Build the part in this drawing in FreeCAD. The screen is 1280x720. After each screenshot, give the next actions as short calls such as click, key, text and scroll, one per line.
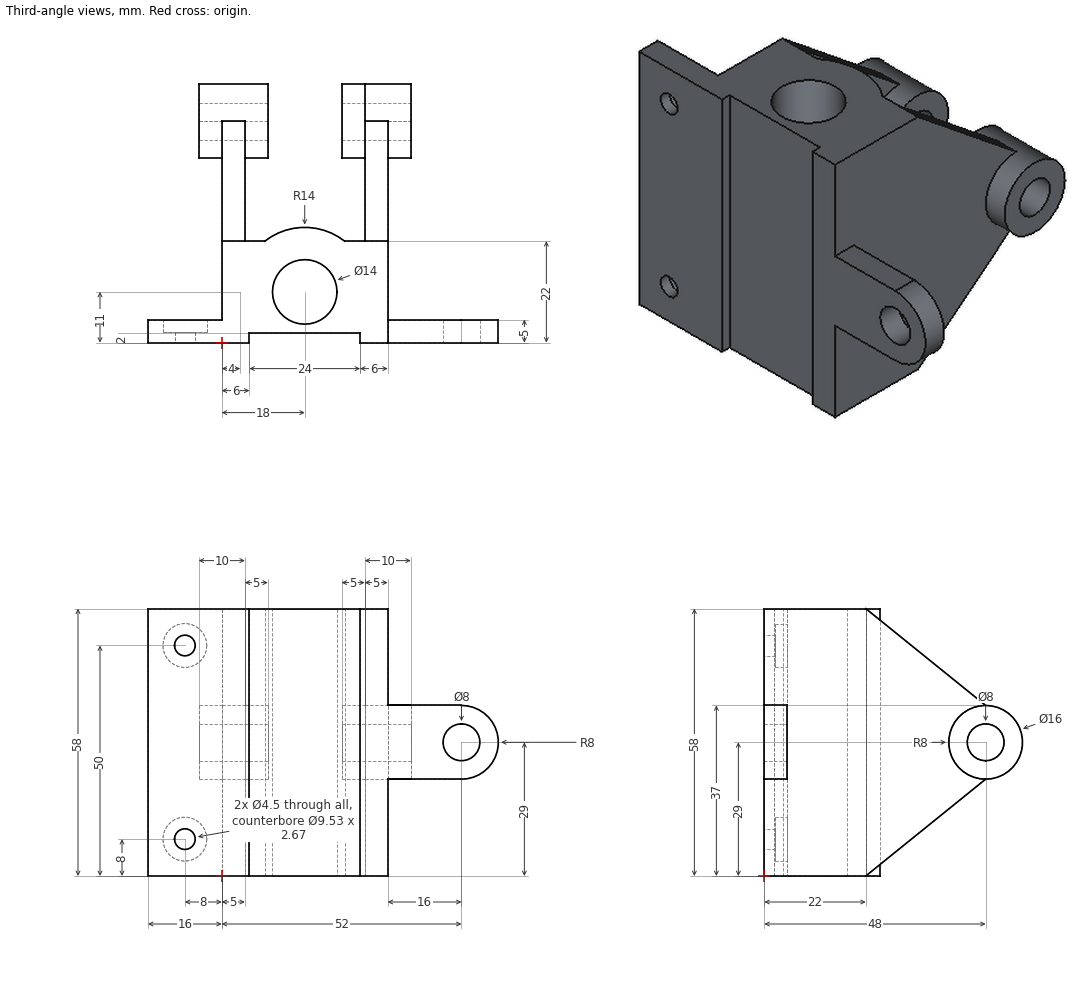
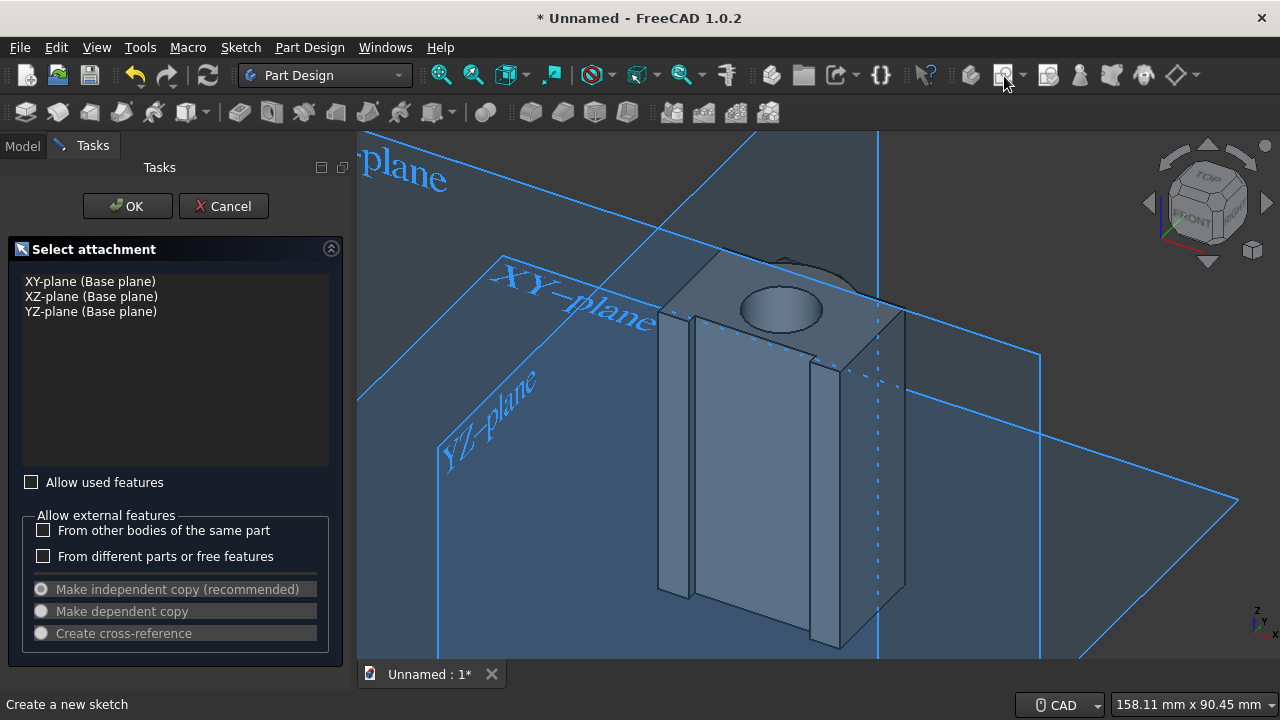
click(82, 312)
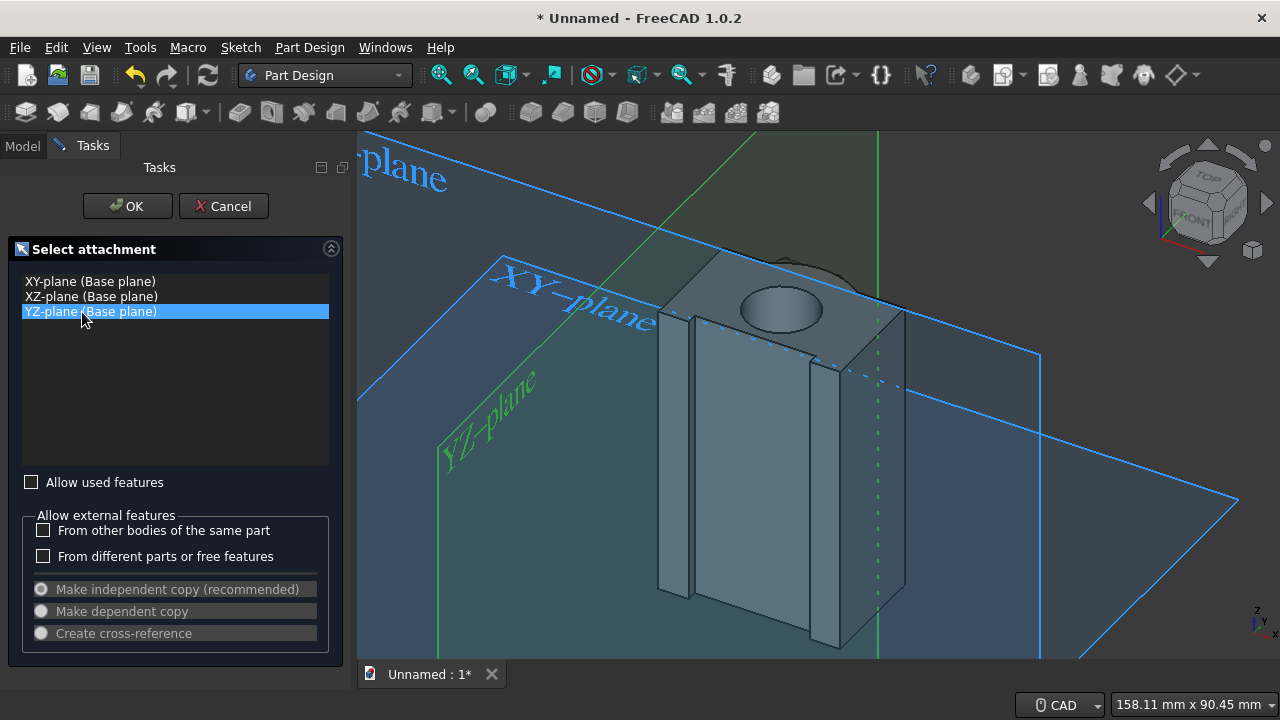
click(128, 206)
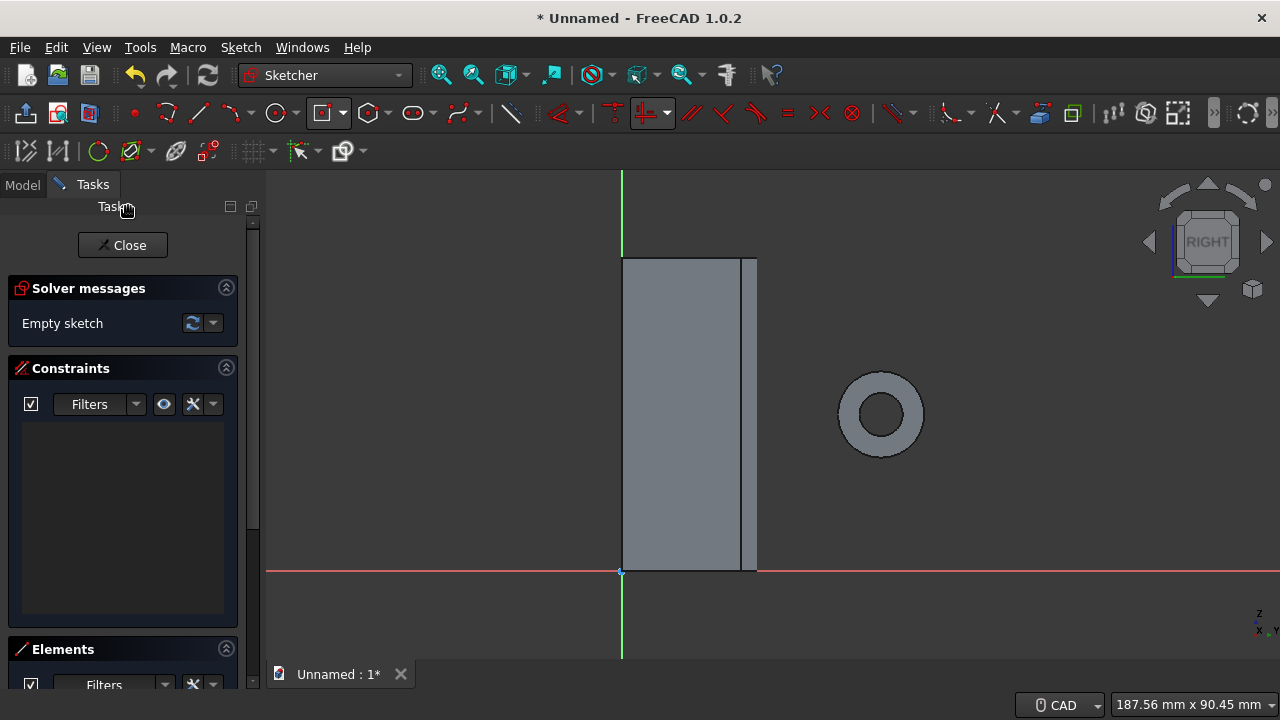
key(q)
key(s)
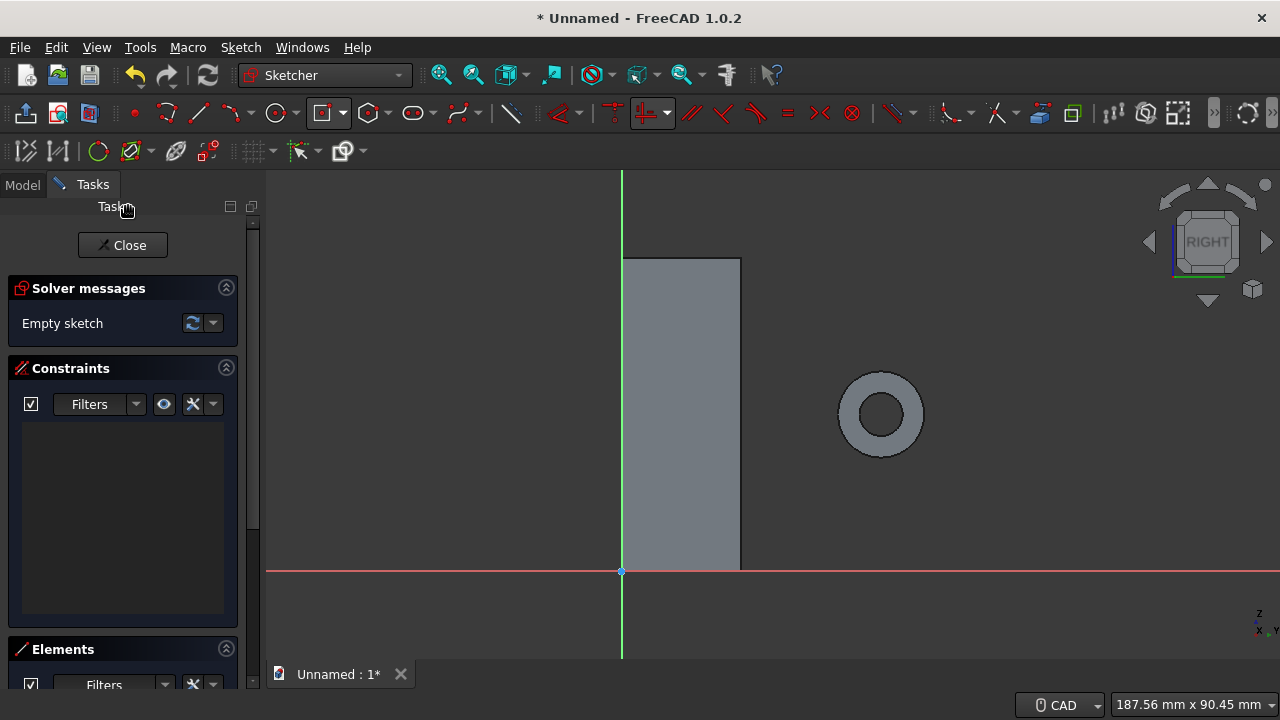
click(168, 114)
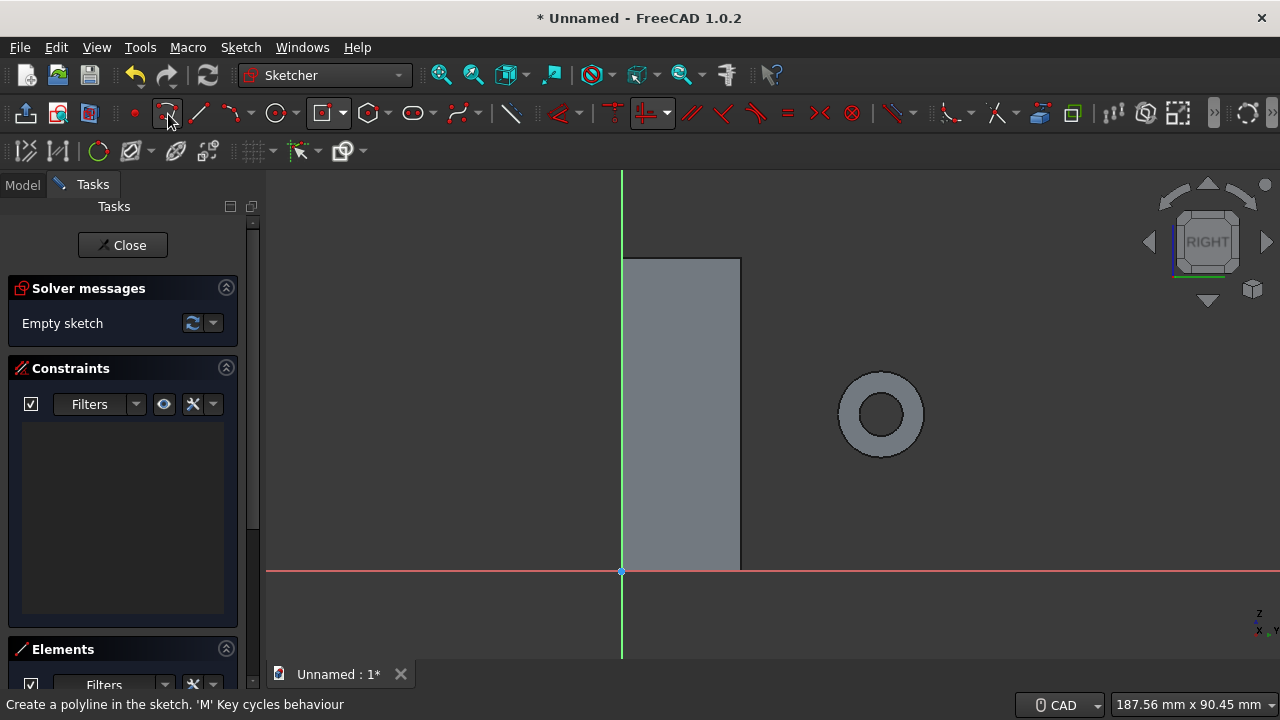
click(881, 371)
click(741, 258)
click(741, 571)
click(881, 458)
right_click(881, 458)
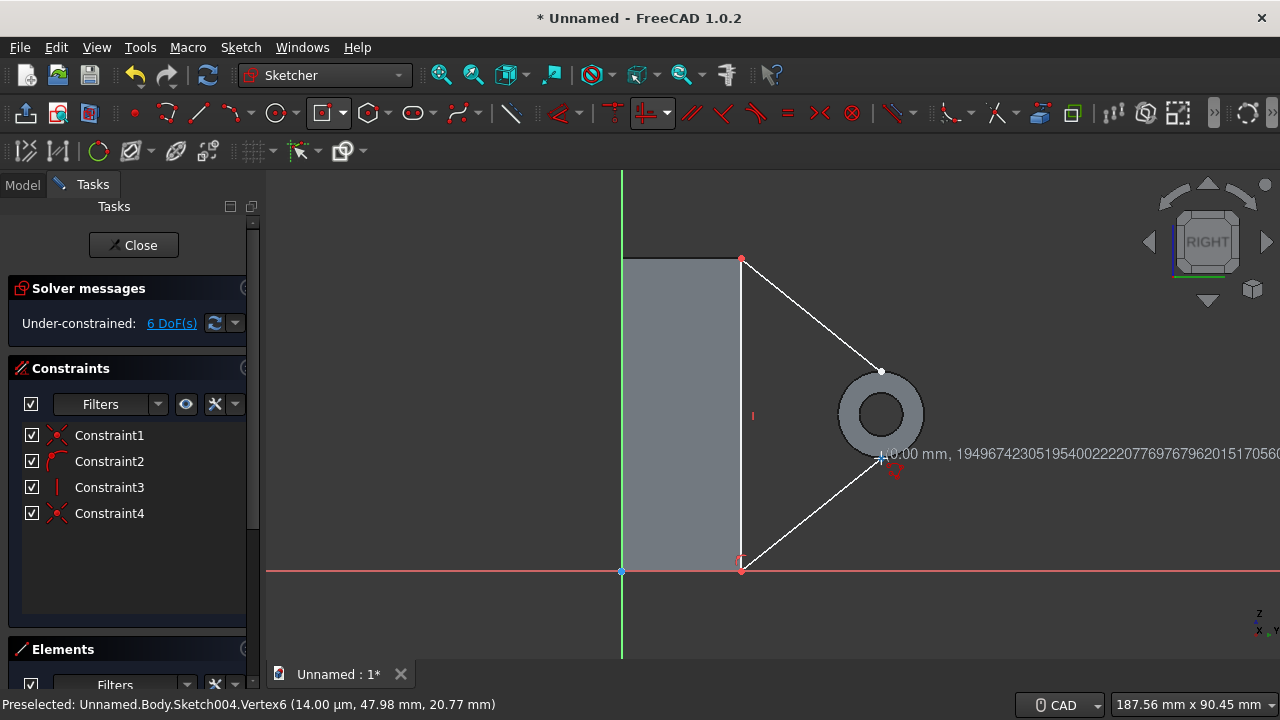
click(232, 114)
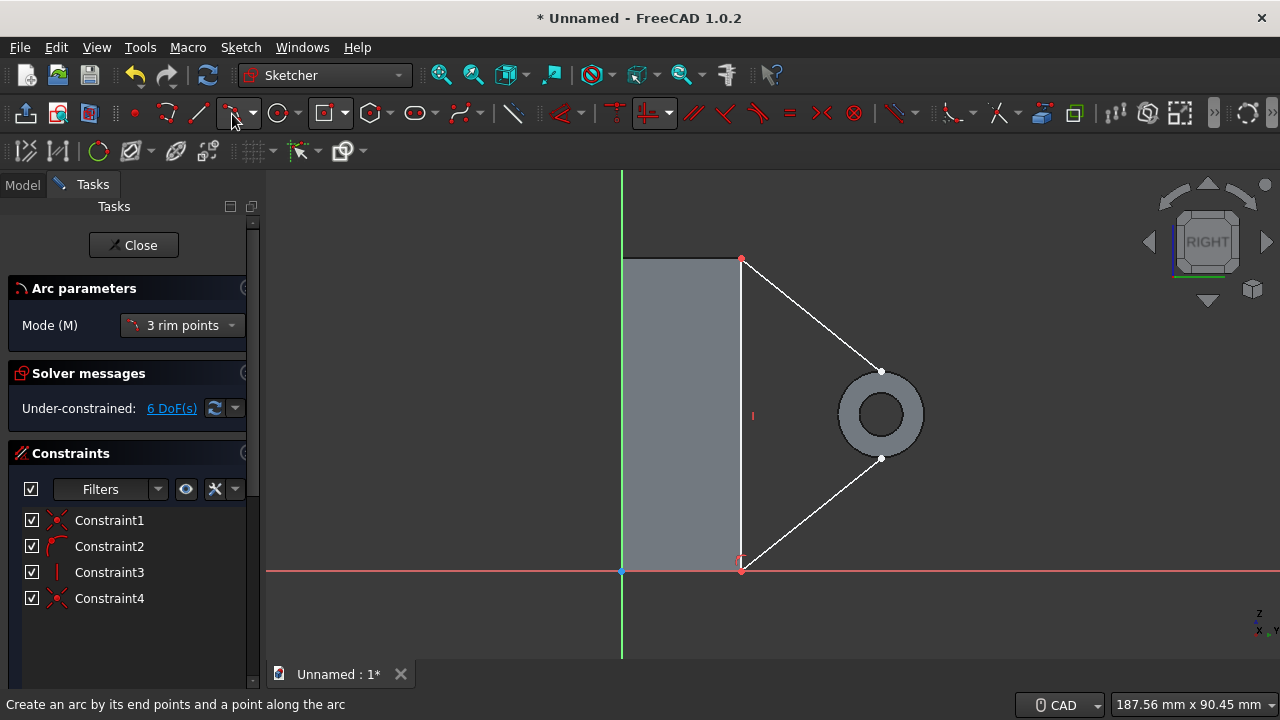
click(881, 459)
click(881, 372)
click(838, 414)
key(Escape)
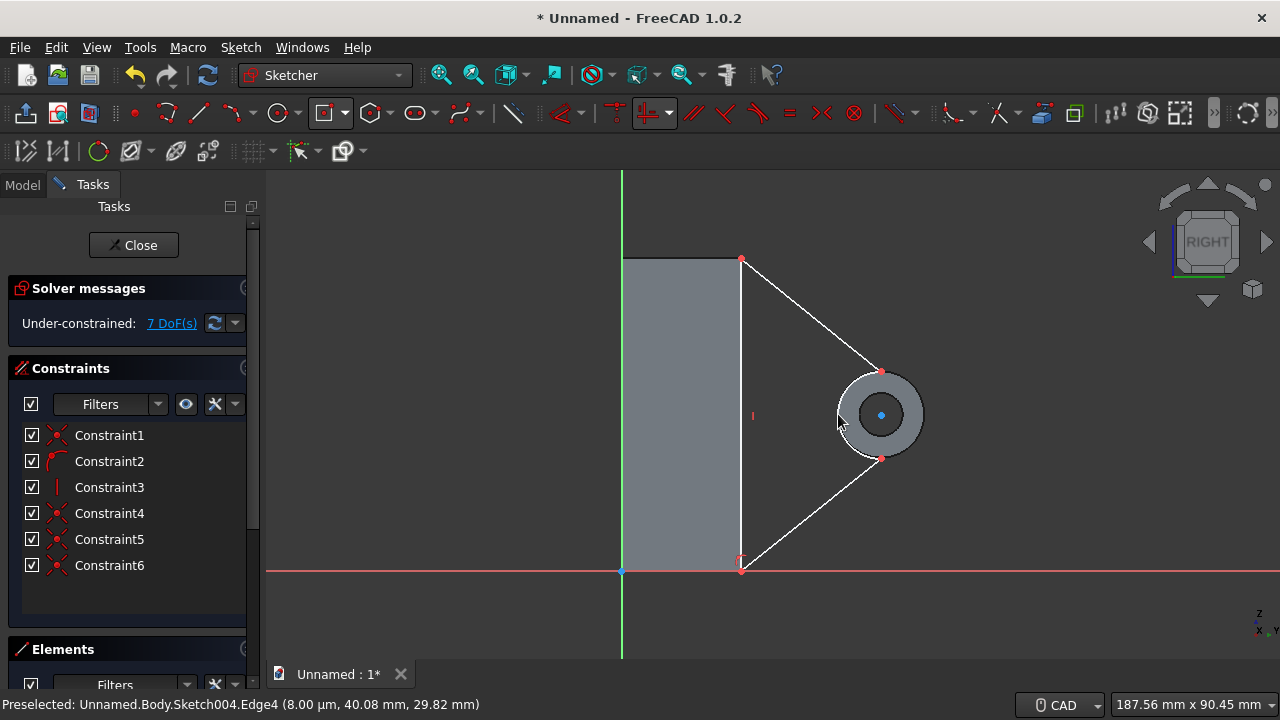
click(560, 114)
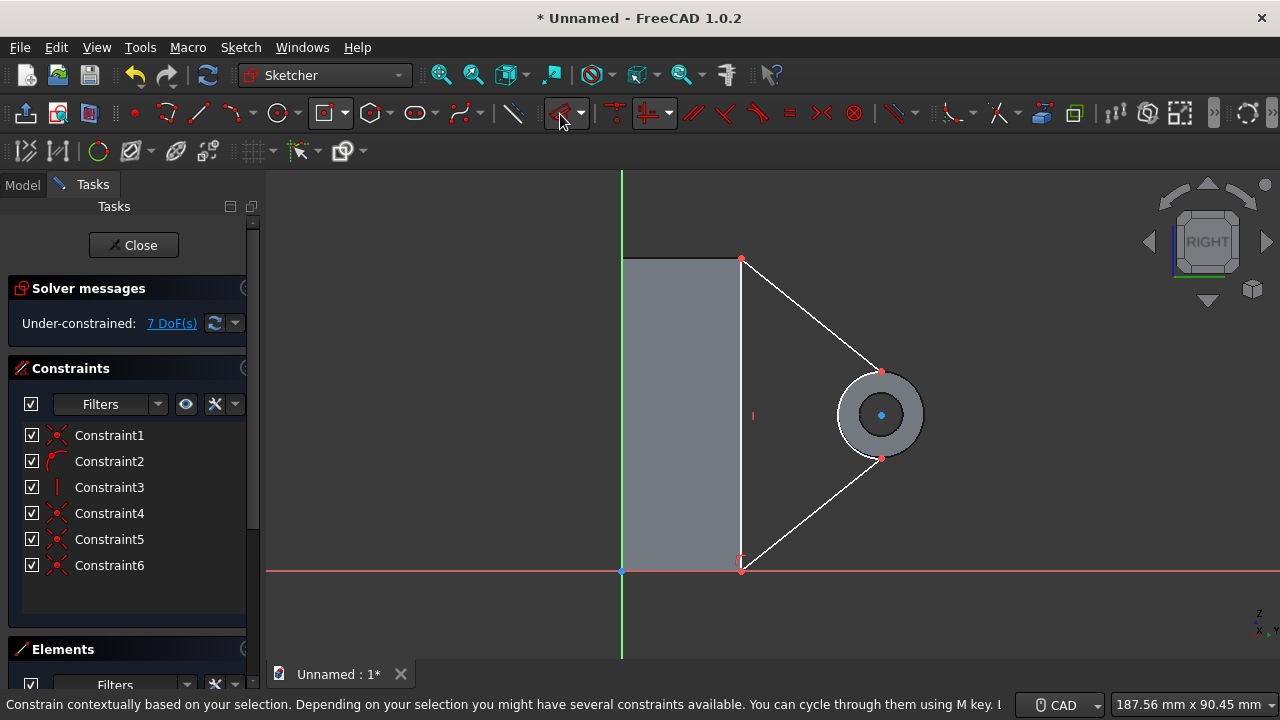
click(846, 390)
click(820, 371)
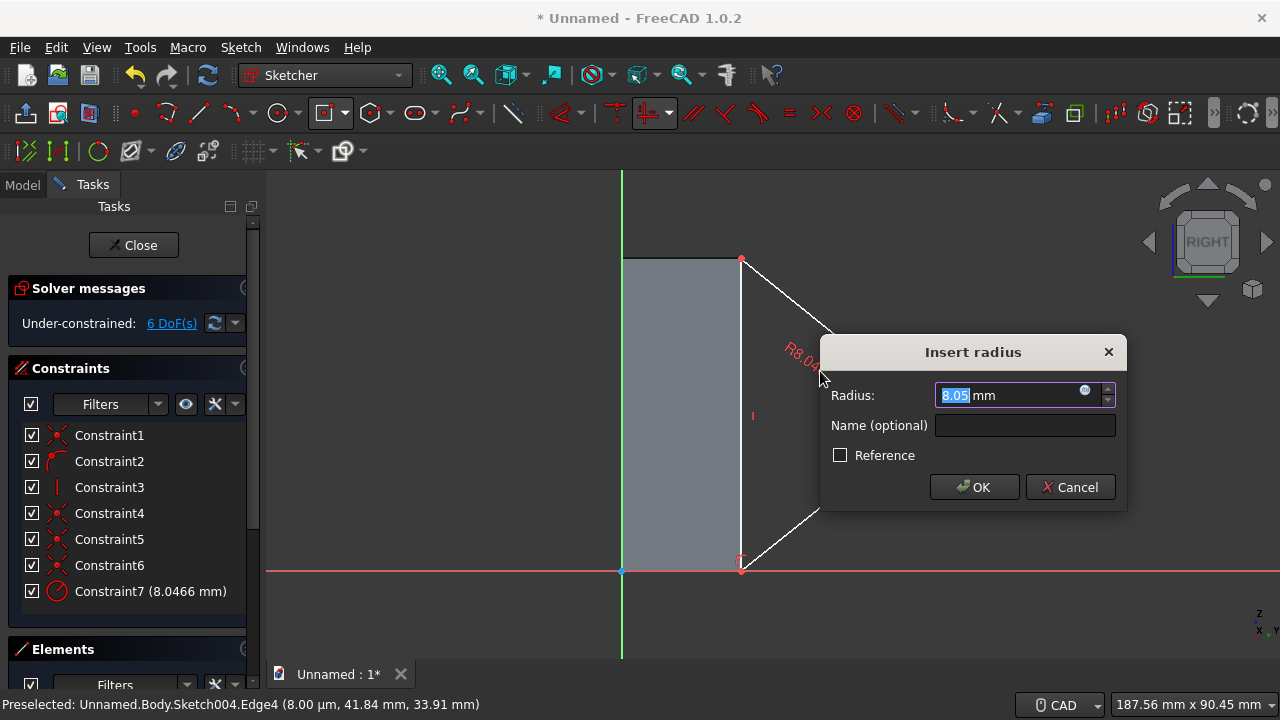
text(8)
key(Return)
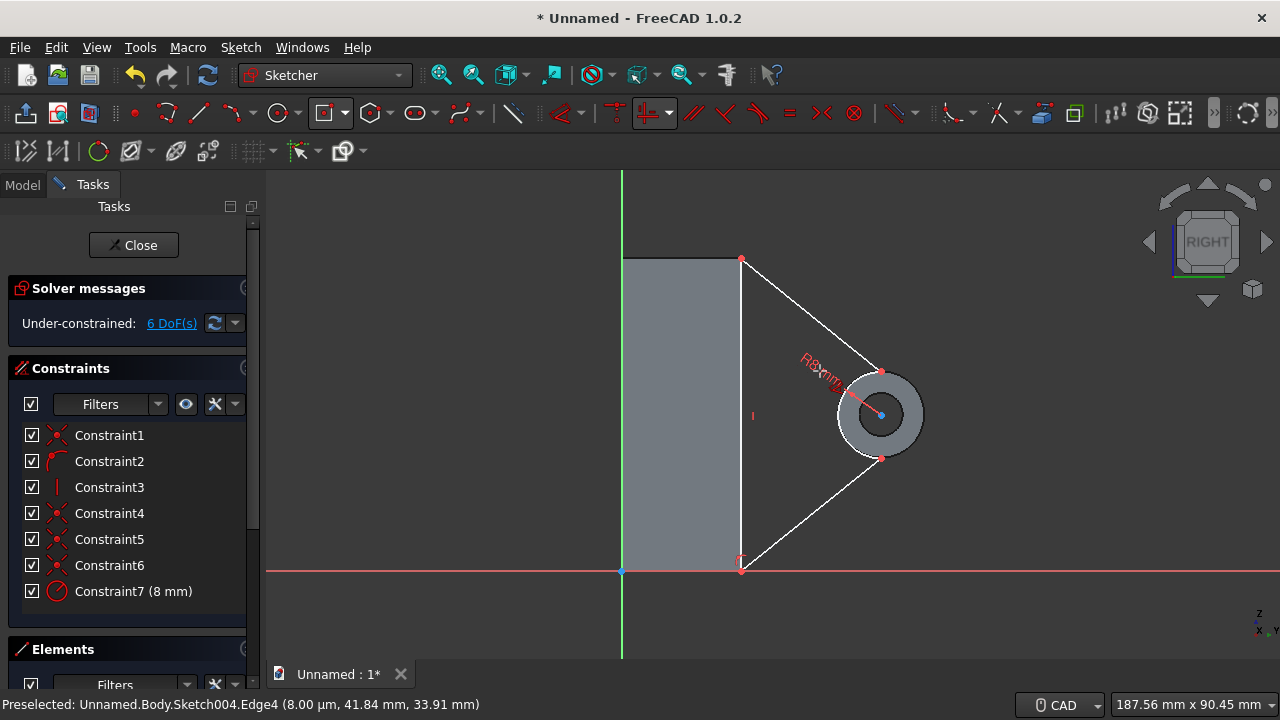
click(741, 353)
click(707, 415)